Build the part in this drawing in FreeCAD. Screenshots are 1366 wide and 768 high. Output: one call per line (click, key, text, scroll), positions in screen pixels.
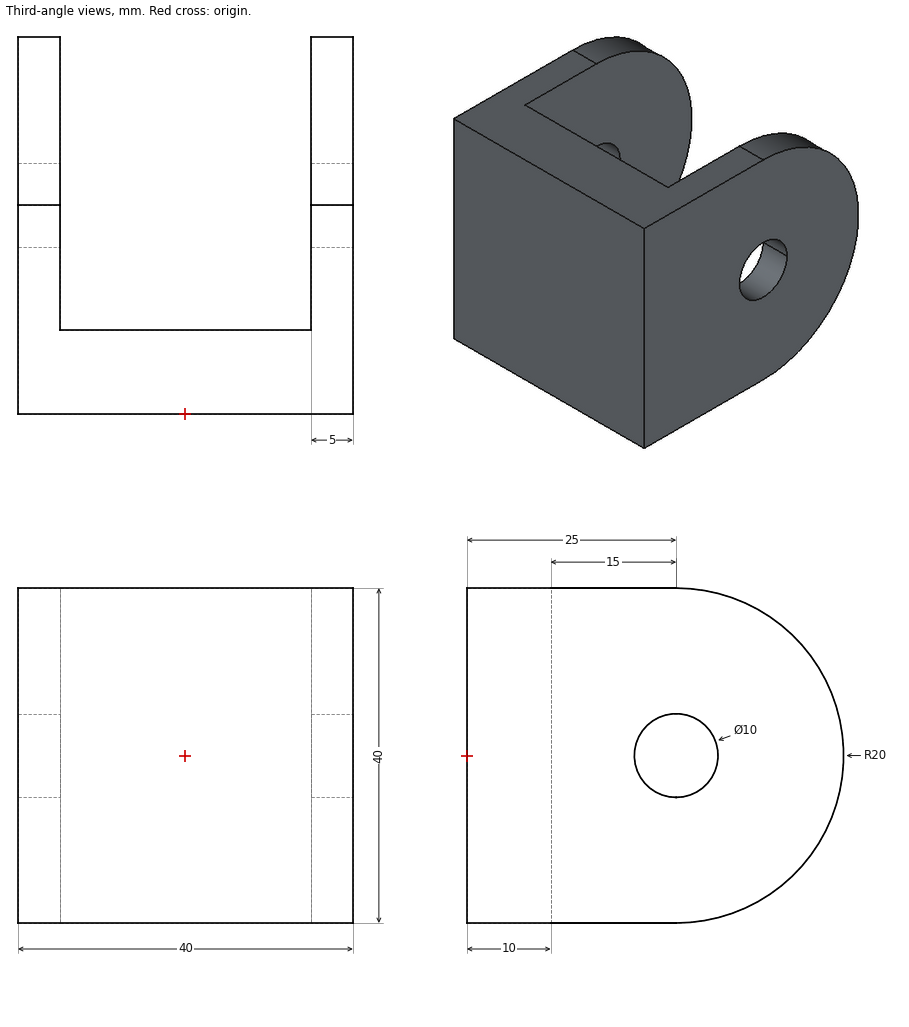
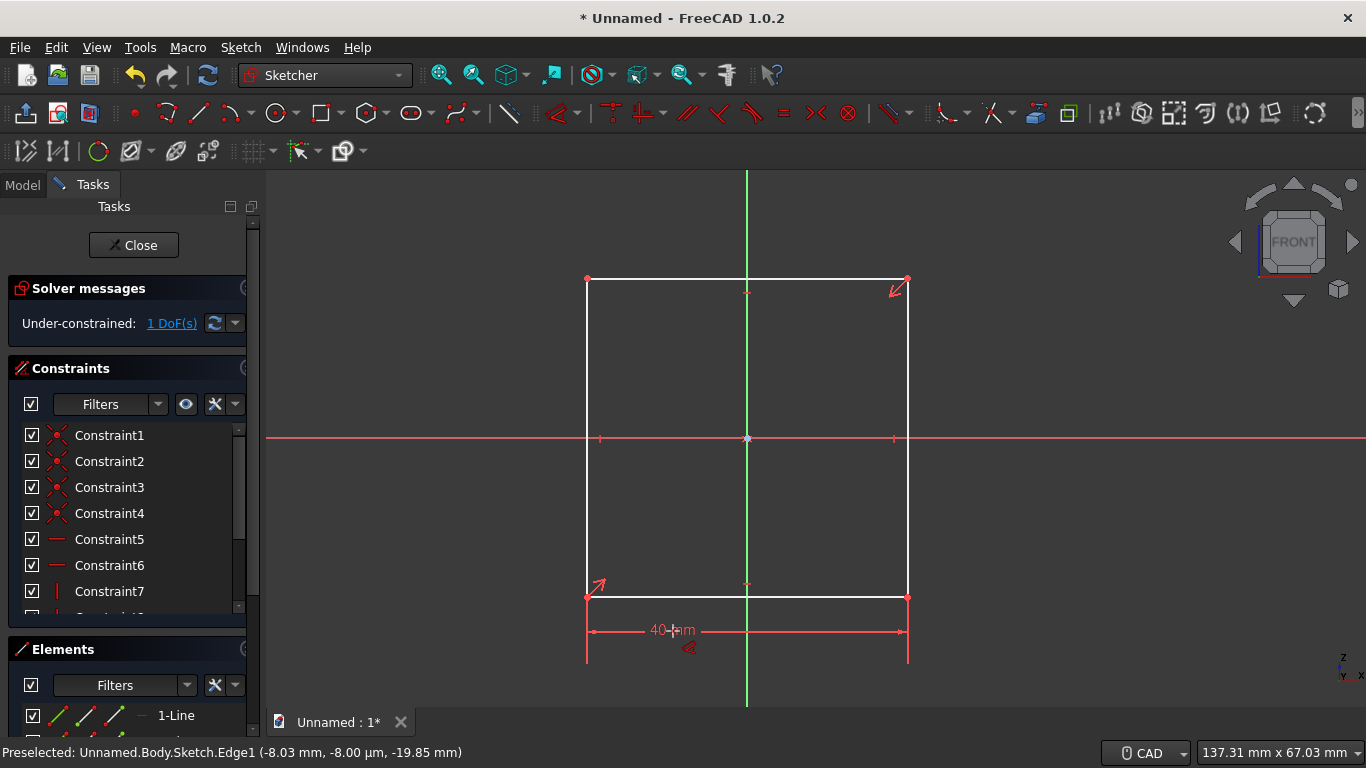
click(908, 502)
click(942, 365)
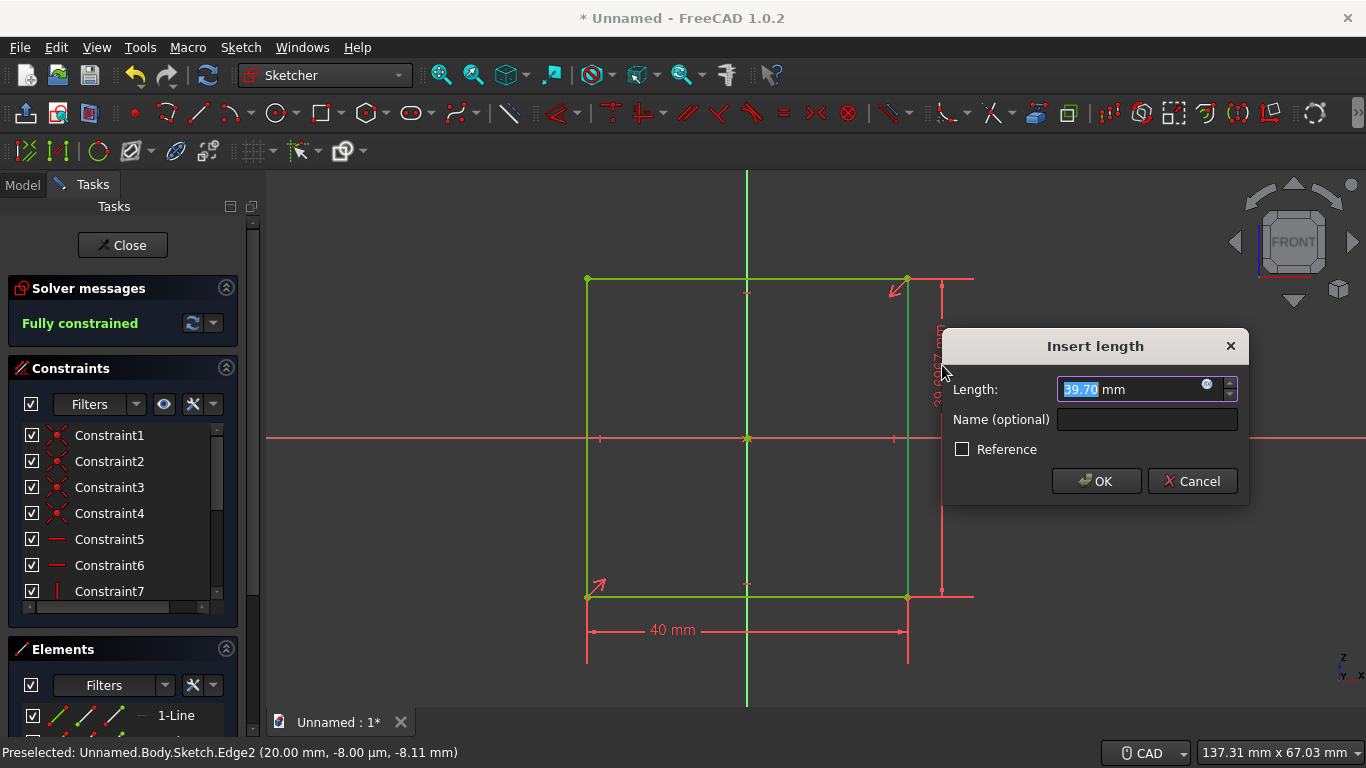
text(40)
key(Return)
key(Escape)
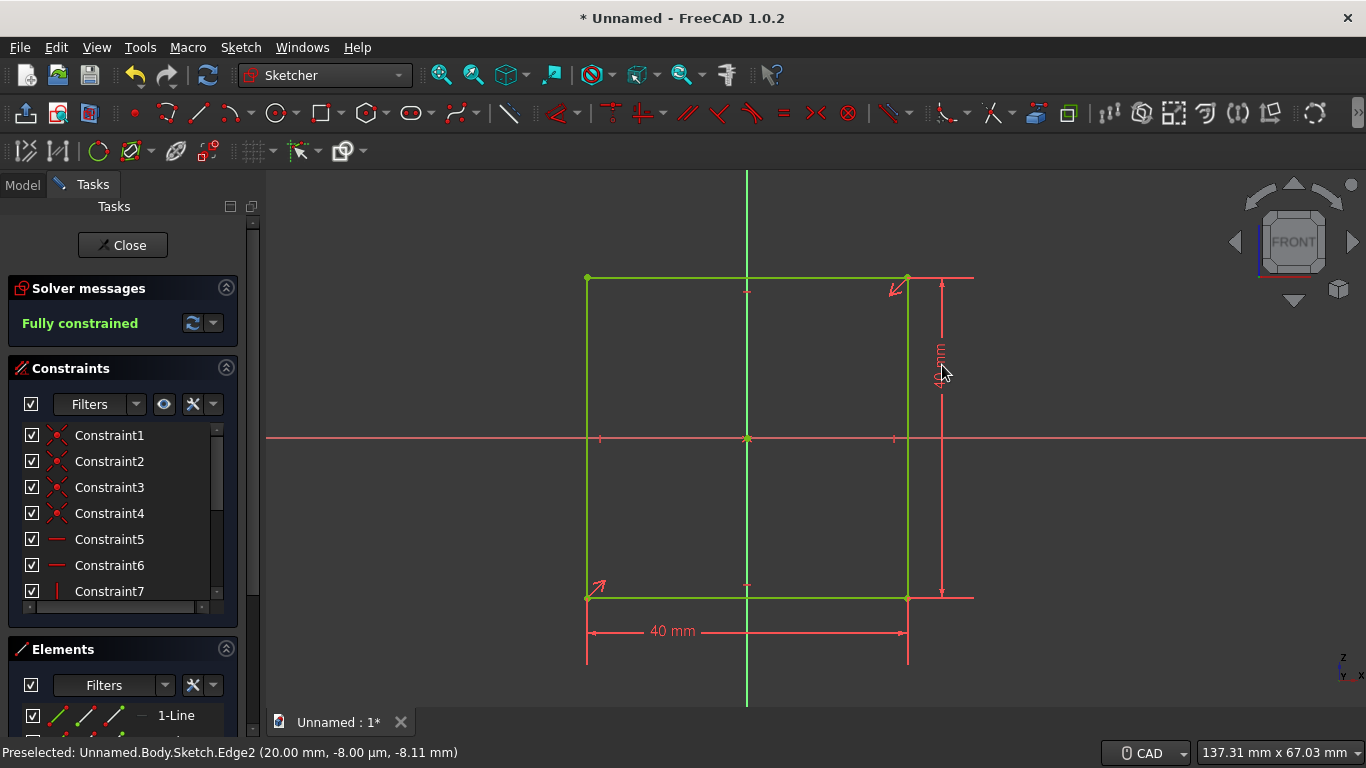
click(123, 245)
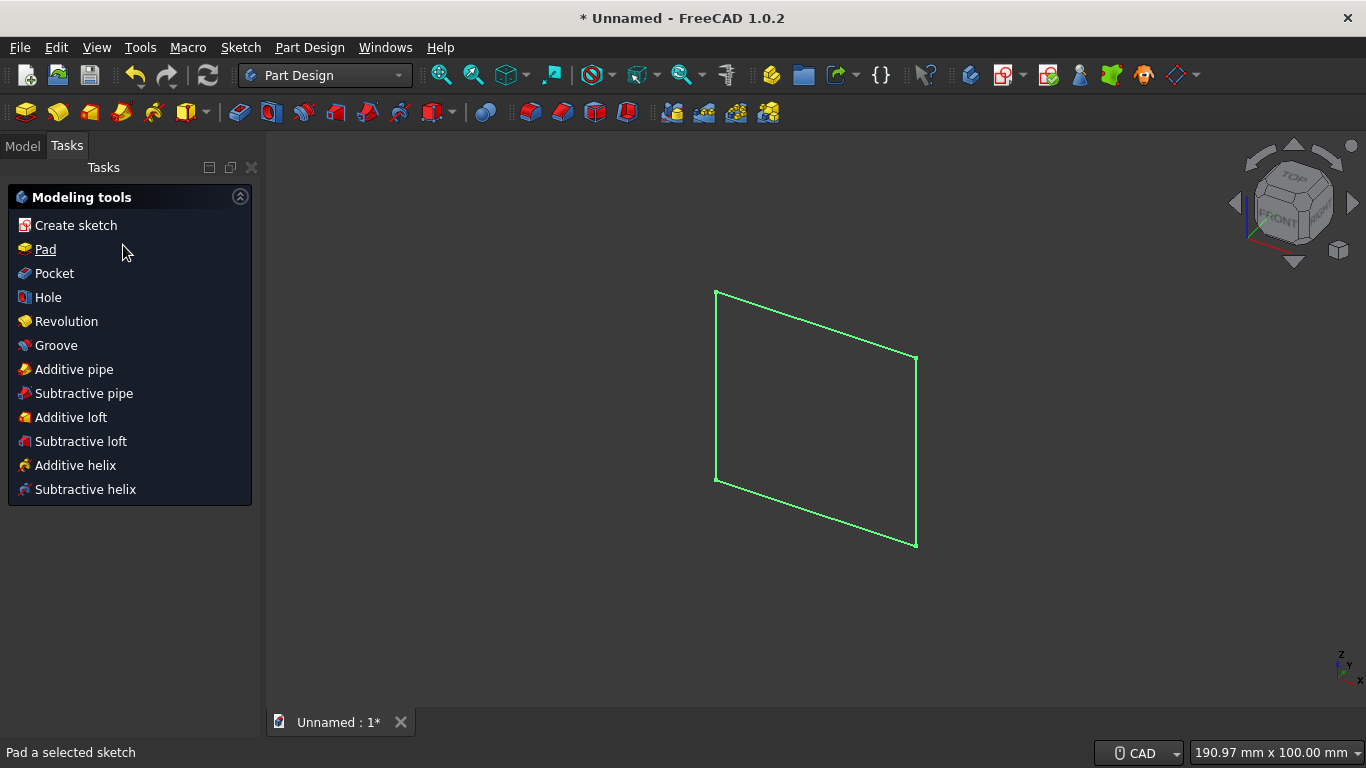
click(26, 112)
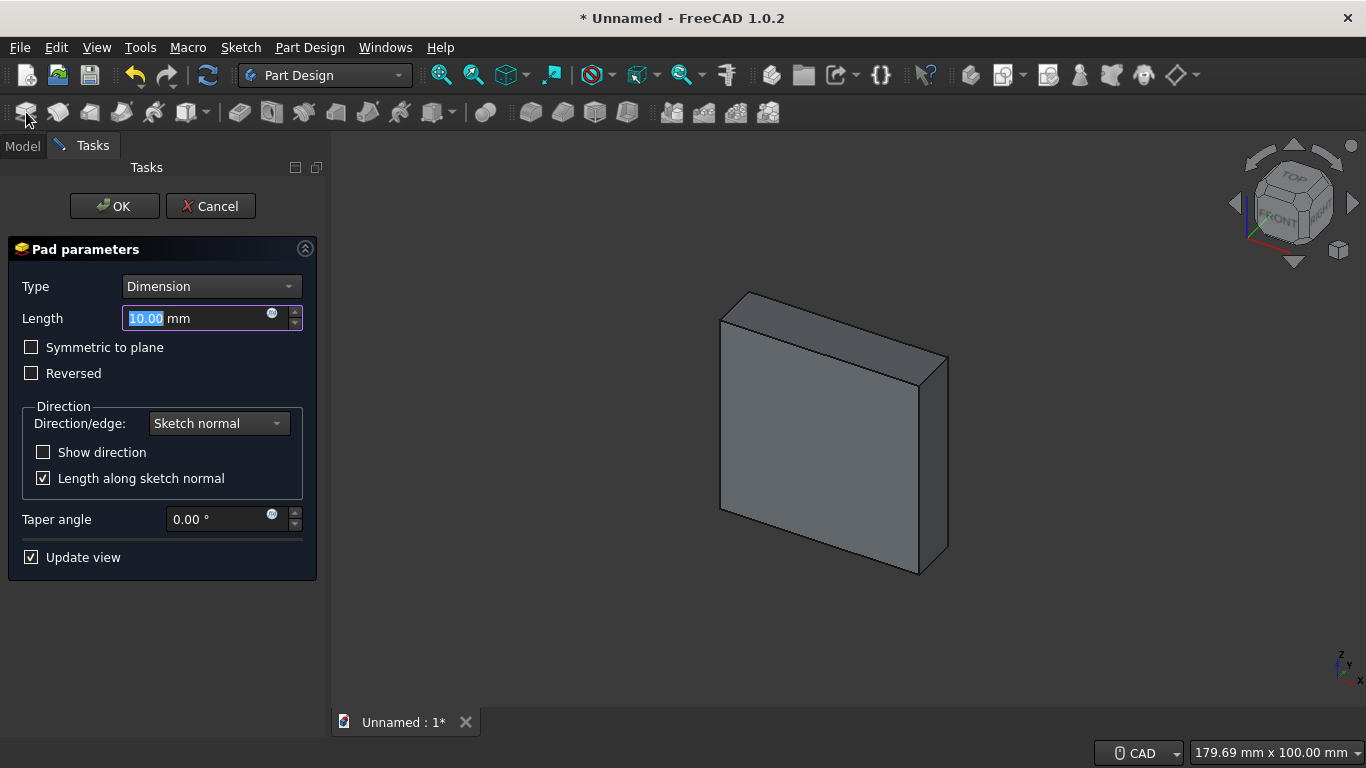
text(10)
key(Tab)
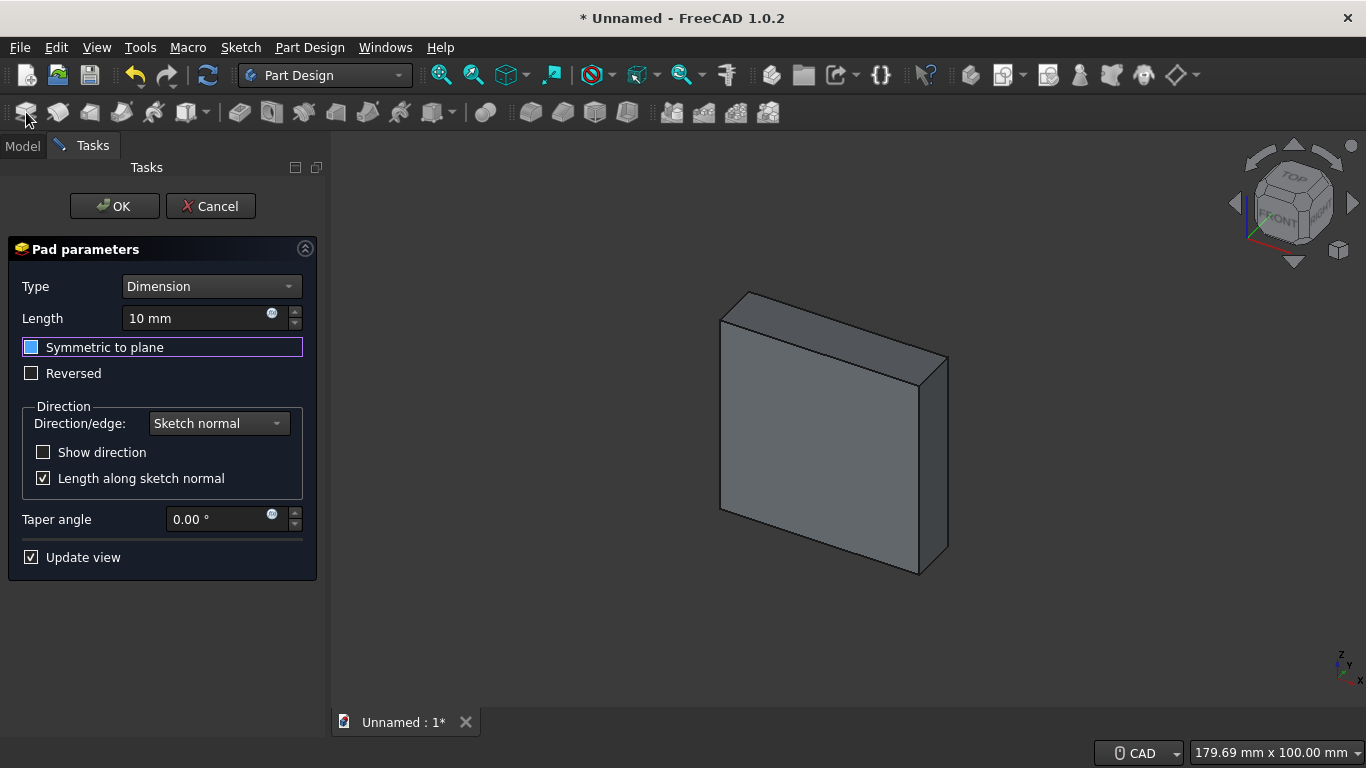
click(30, 373)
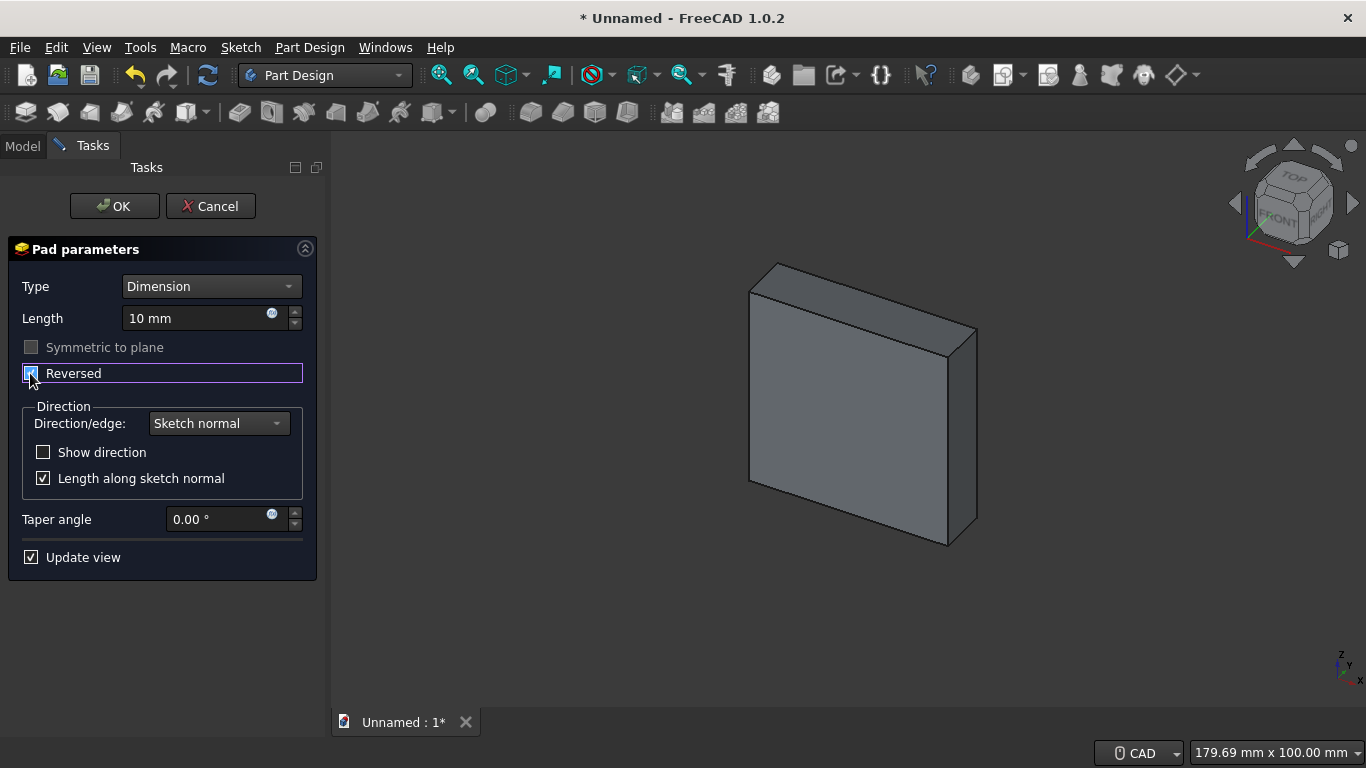
click(115, 206)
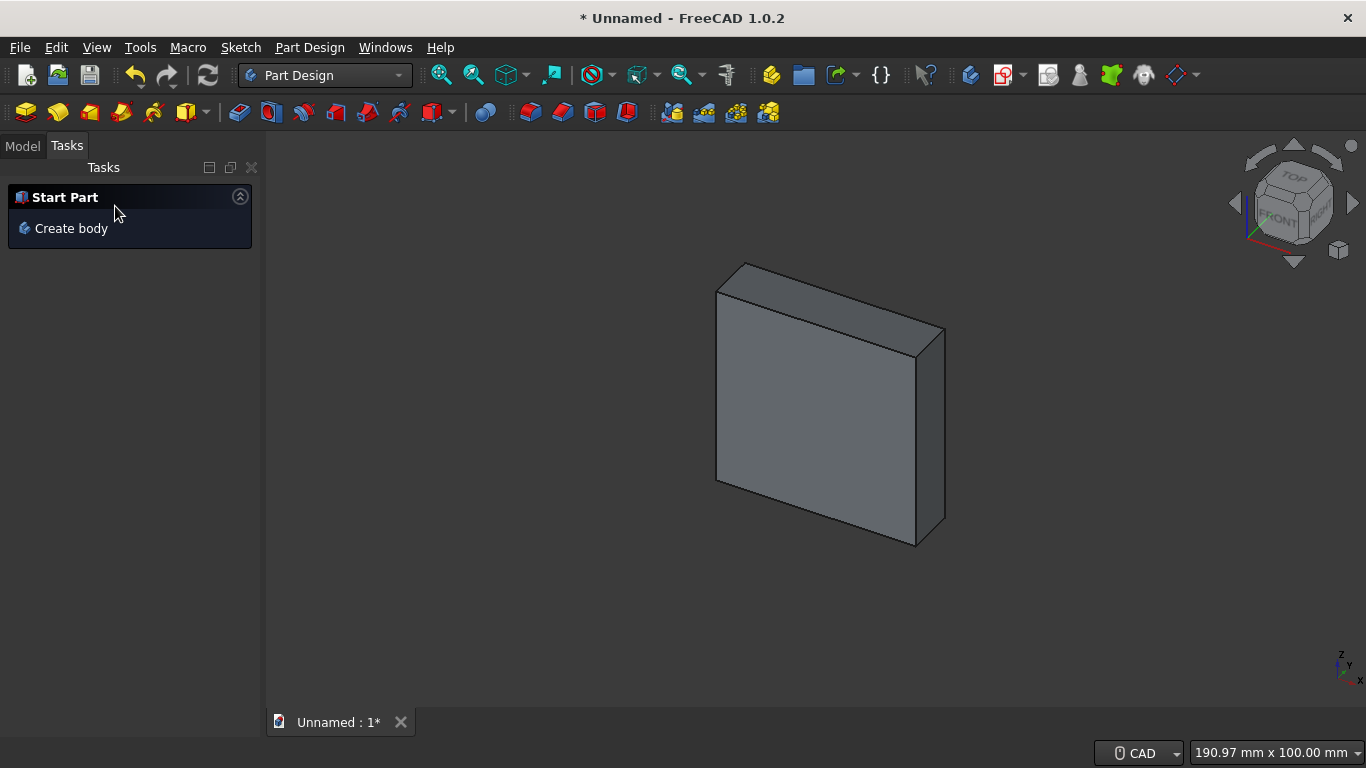
click(930, 437)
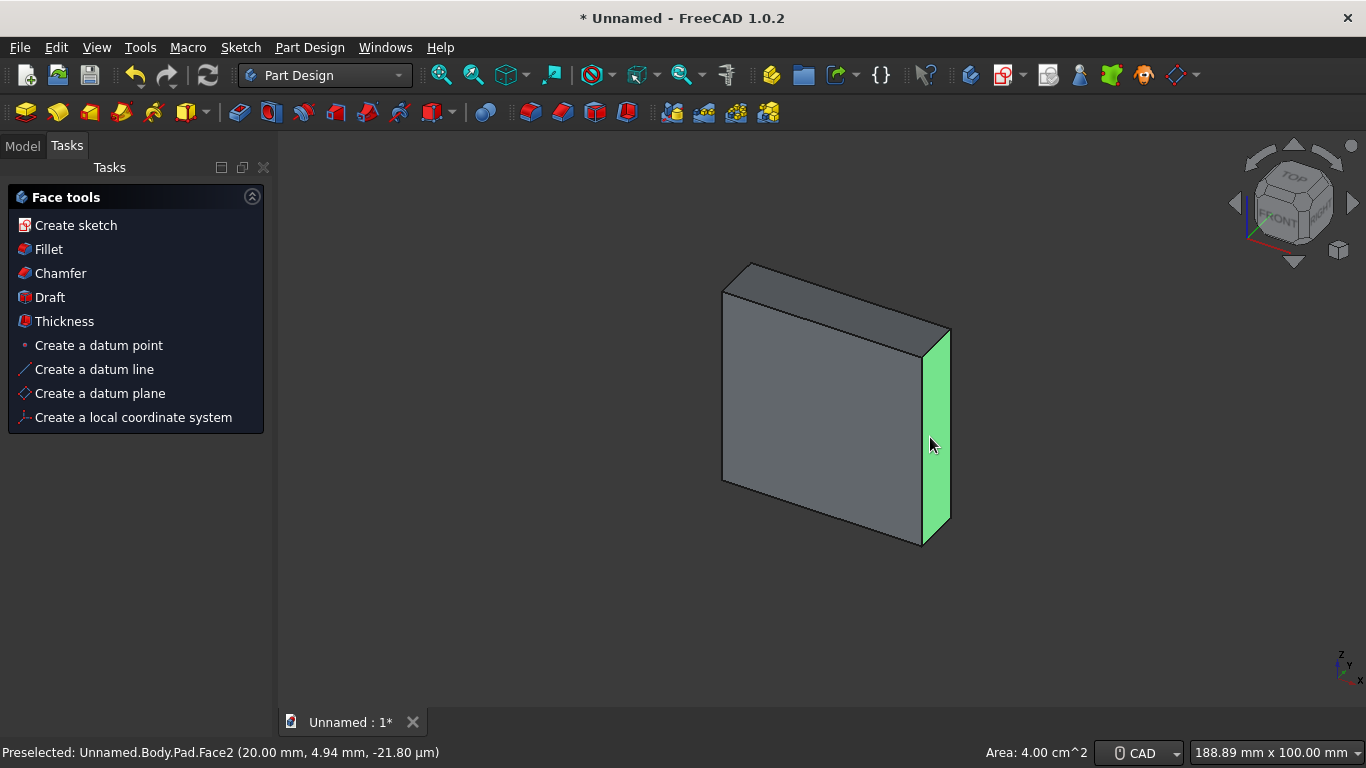
click(1004, 76)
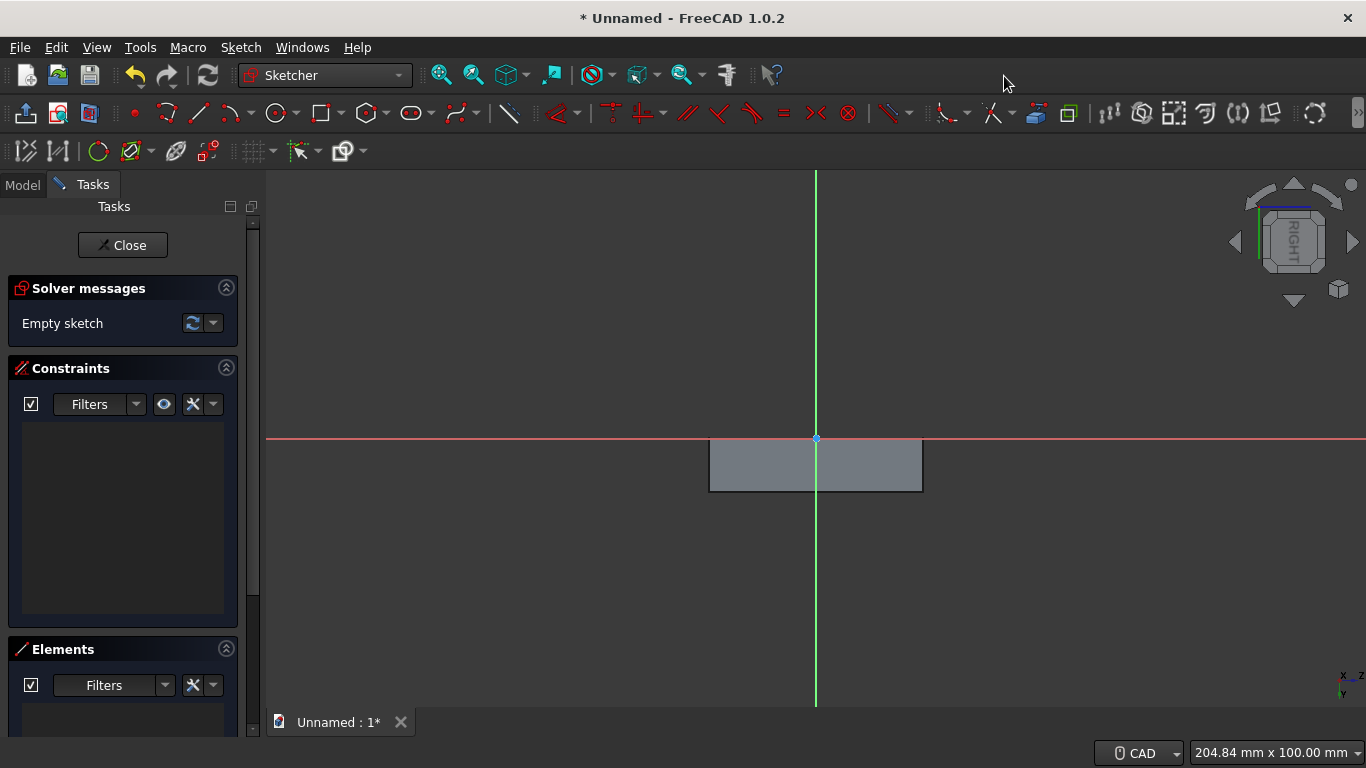
scroll(438, 198, down, 1)